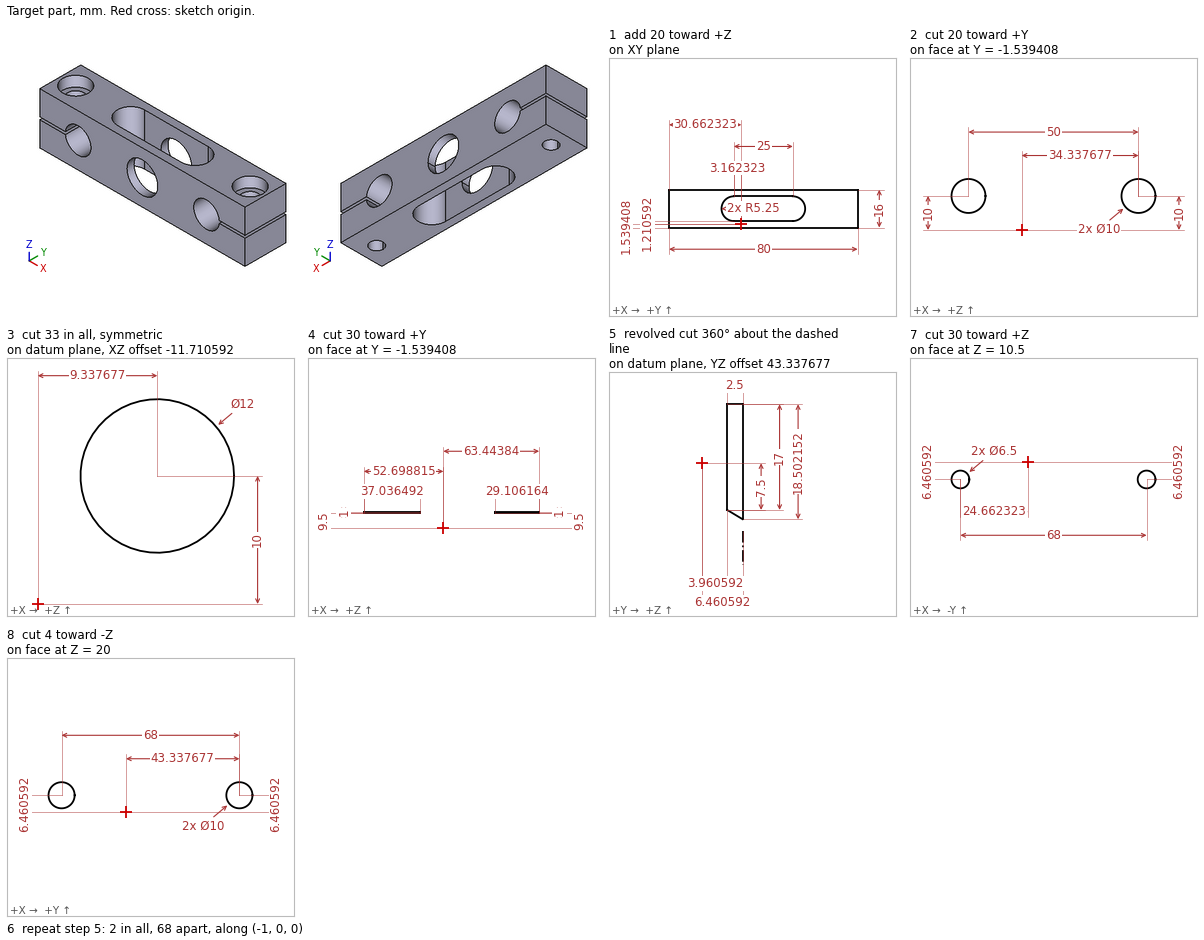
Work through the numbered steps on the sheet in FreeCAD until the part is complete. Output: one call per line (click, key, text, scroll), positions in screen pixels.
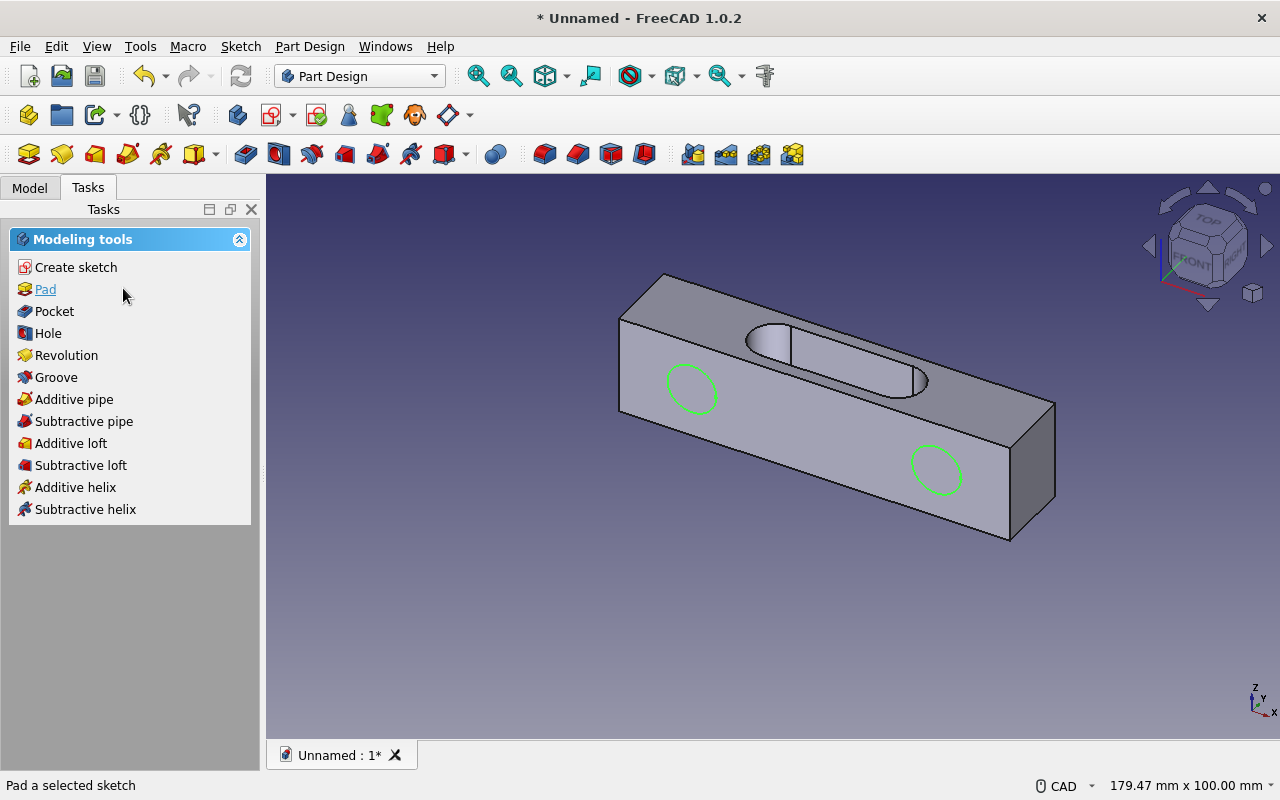
click(246, 154)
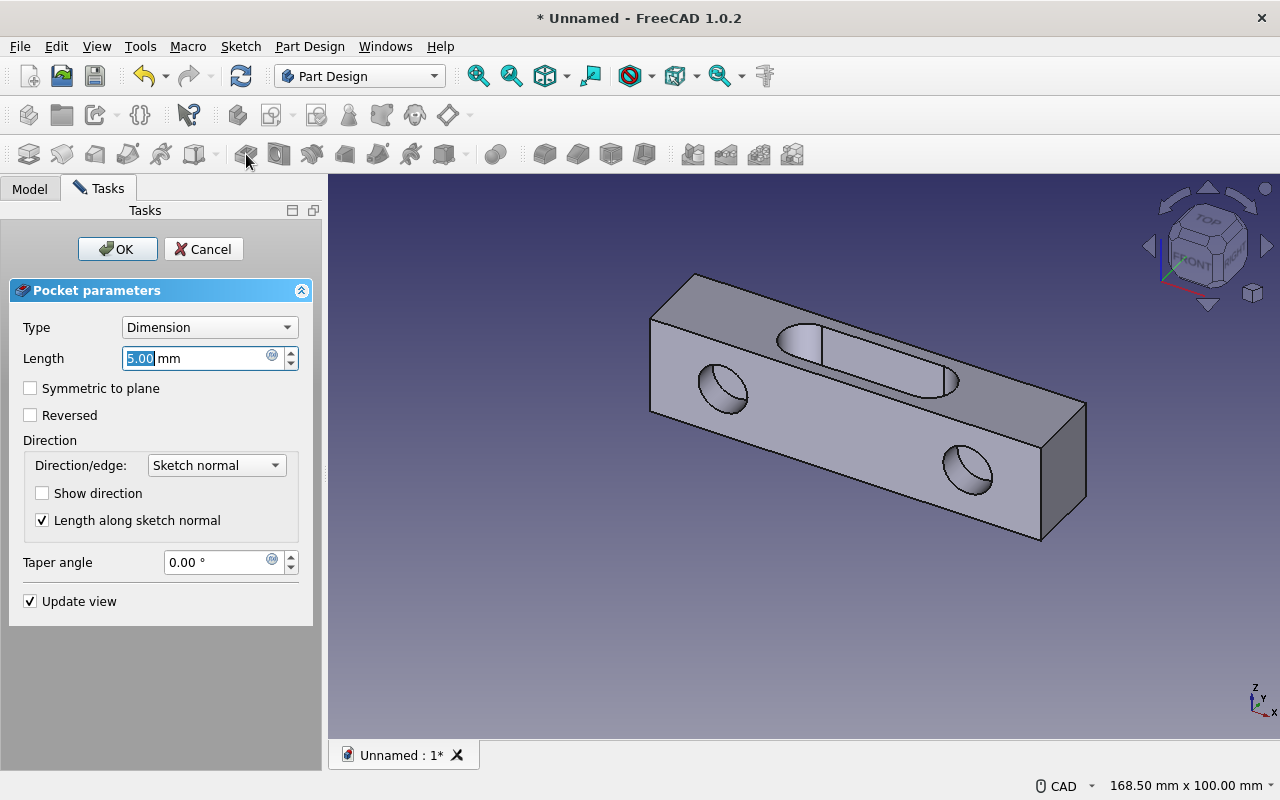
text(20)
key(Tab)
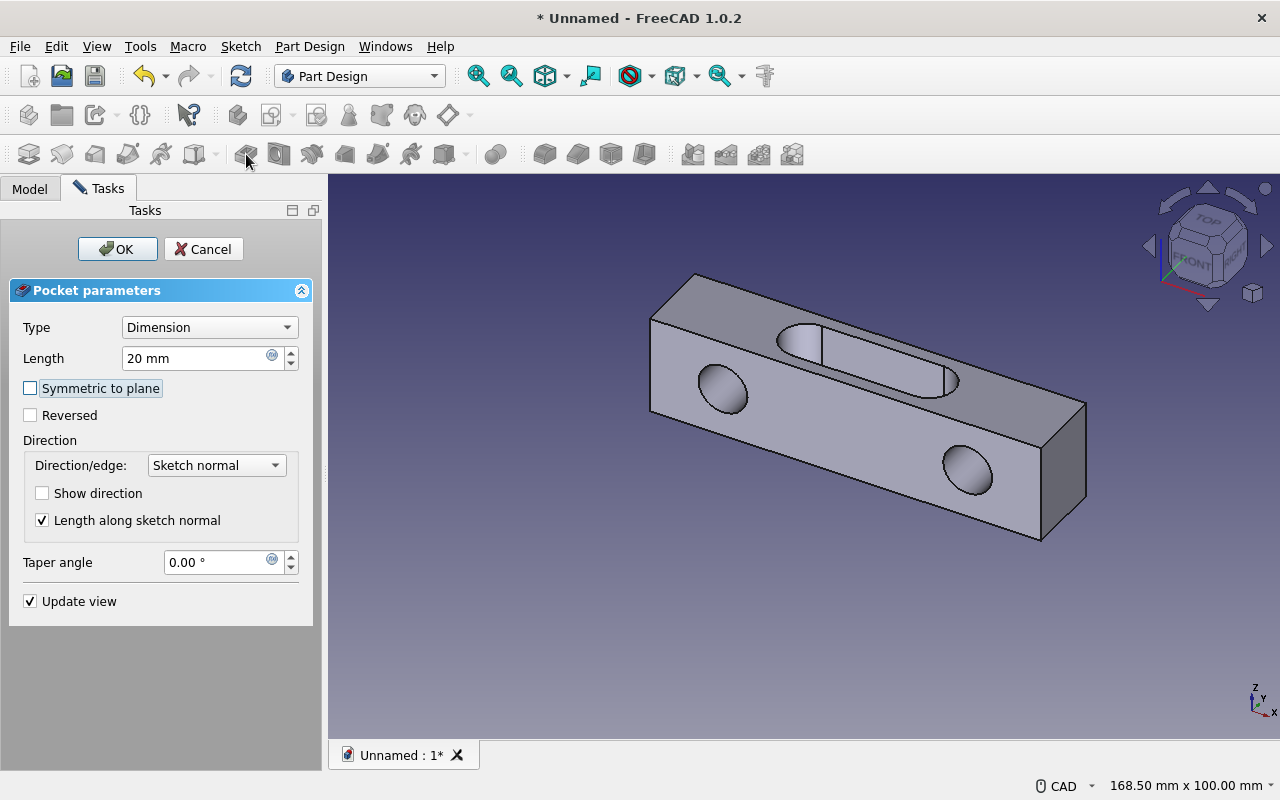
click(118, 249)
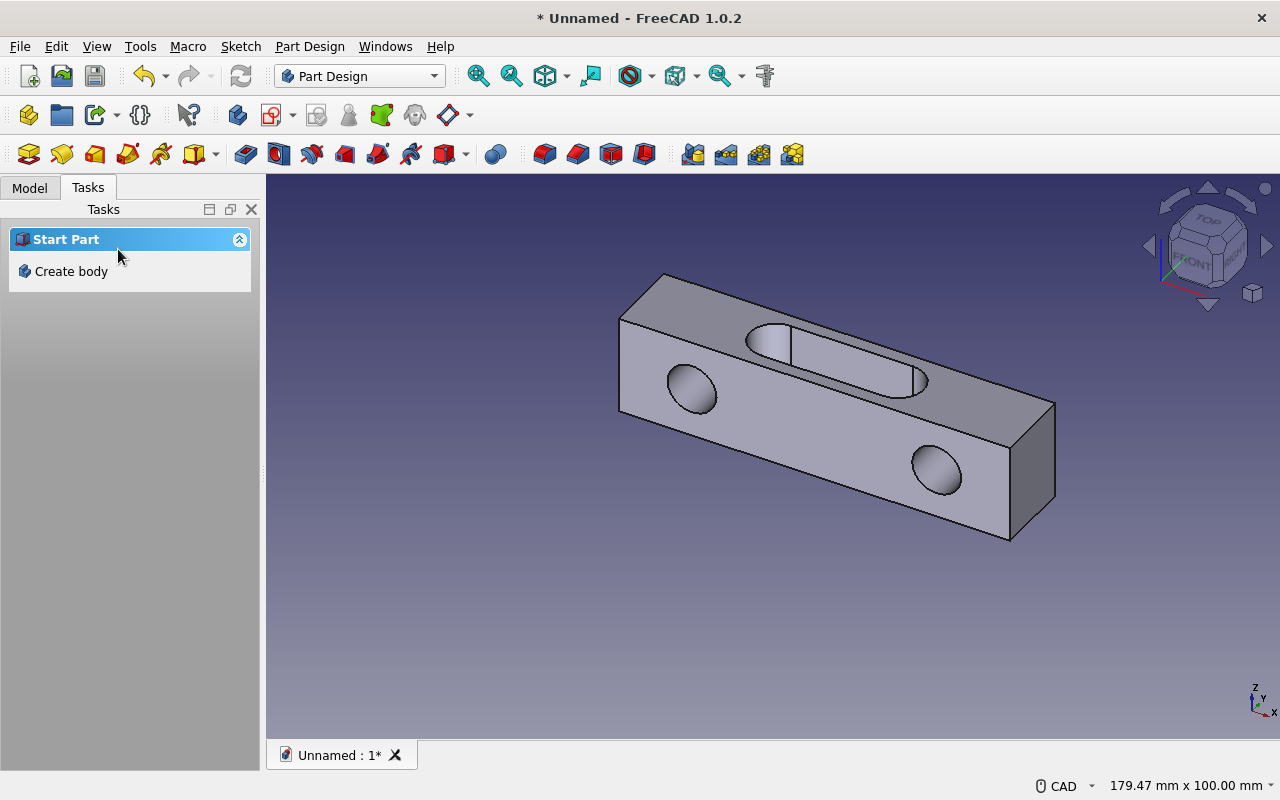
click(30, 188)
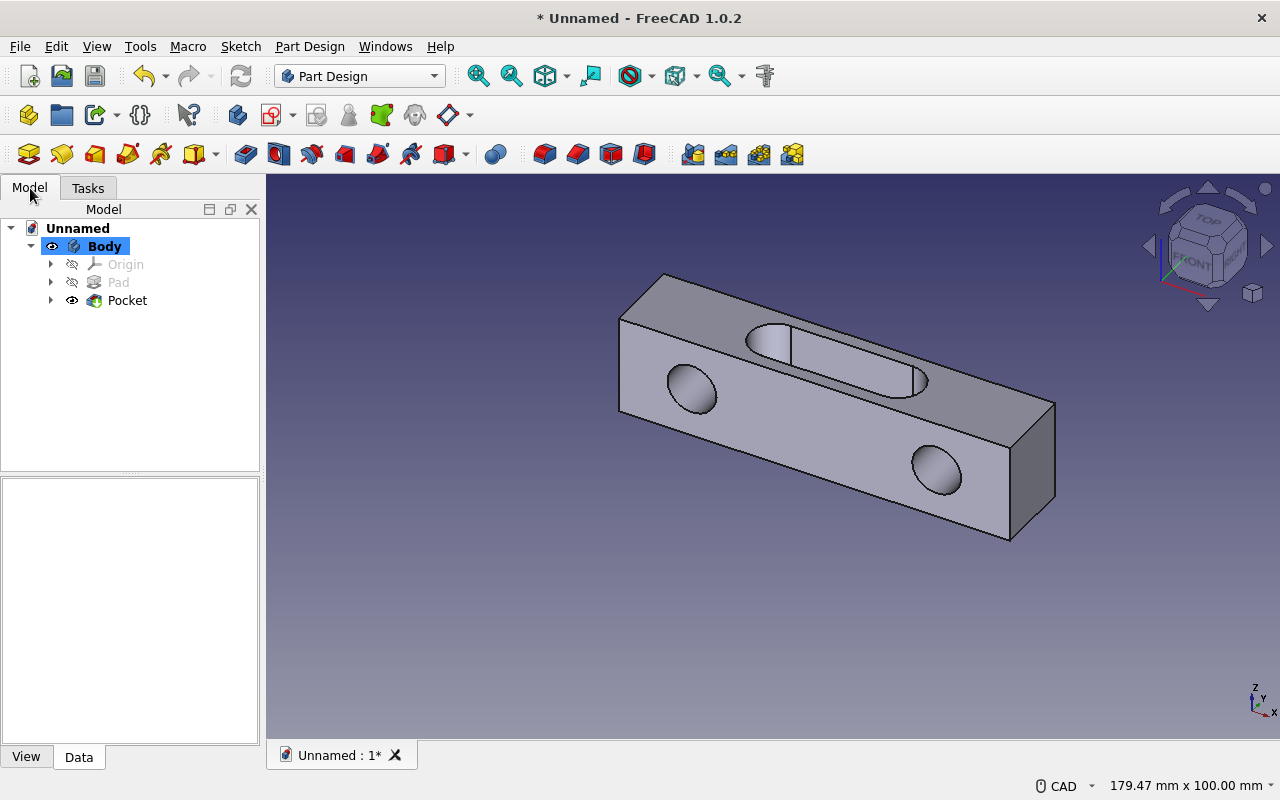
click(51, 264)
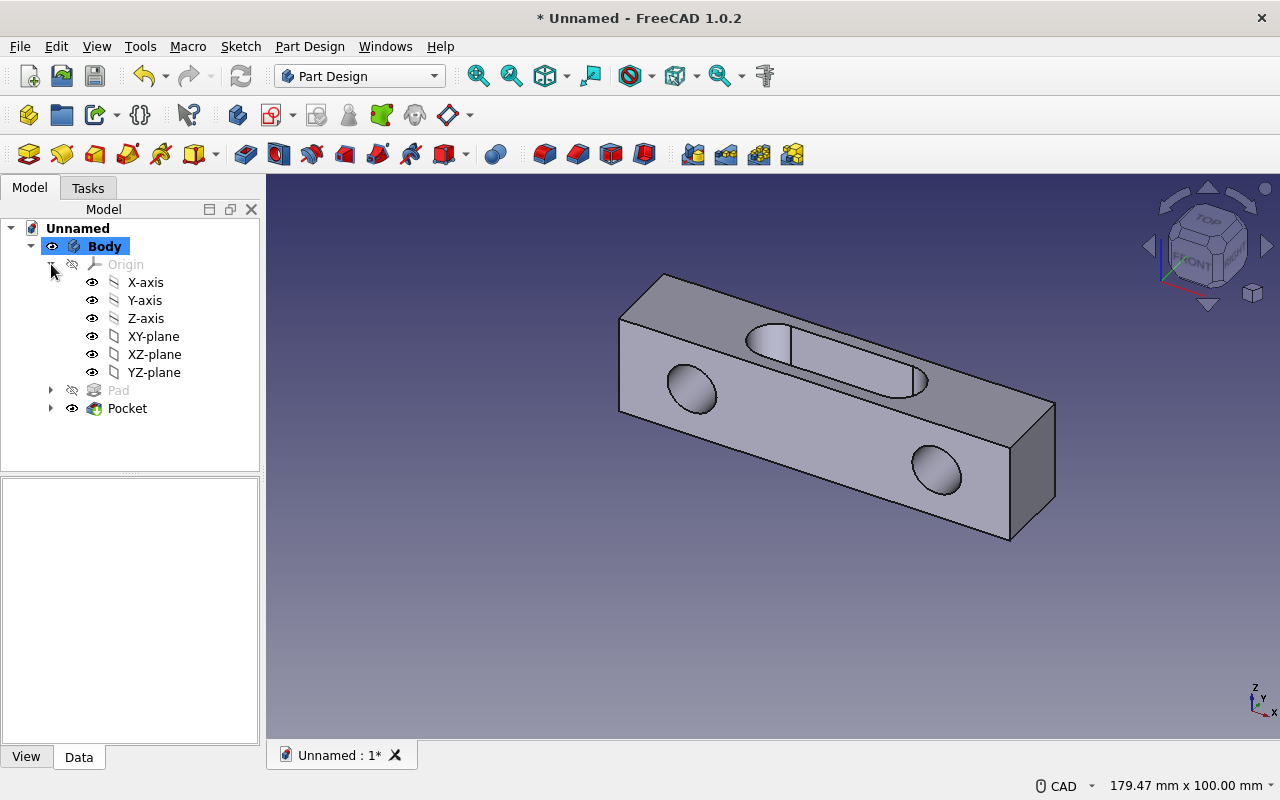
click(137, 354)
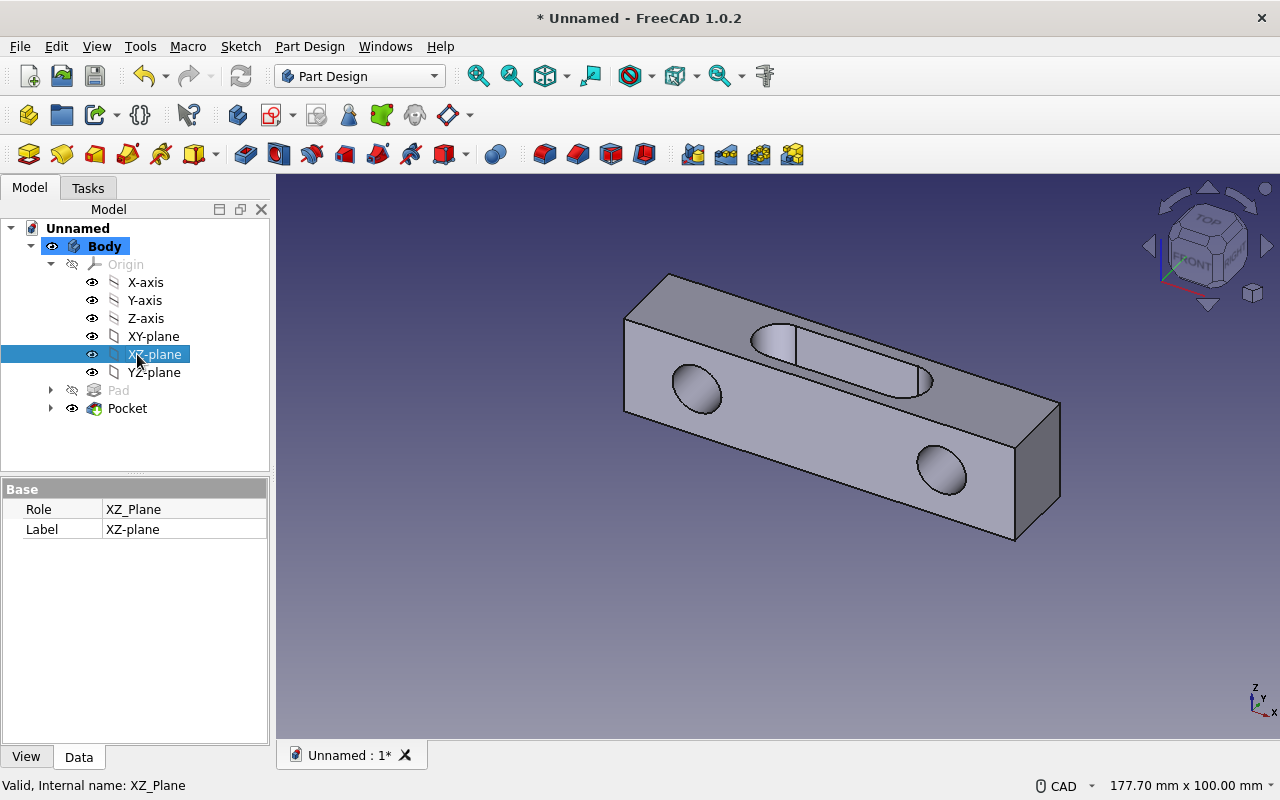
click(448, 116)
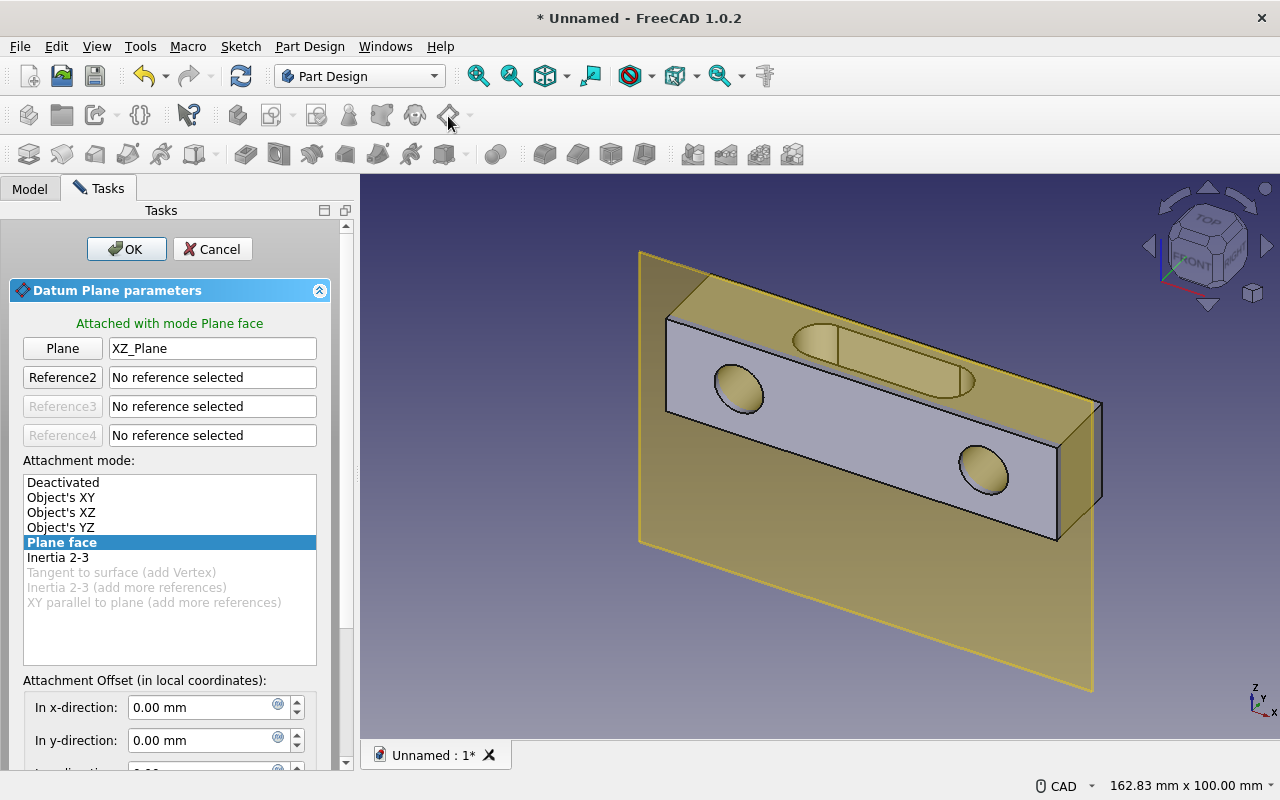
scroll(346, 495, down, 2)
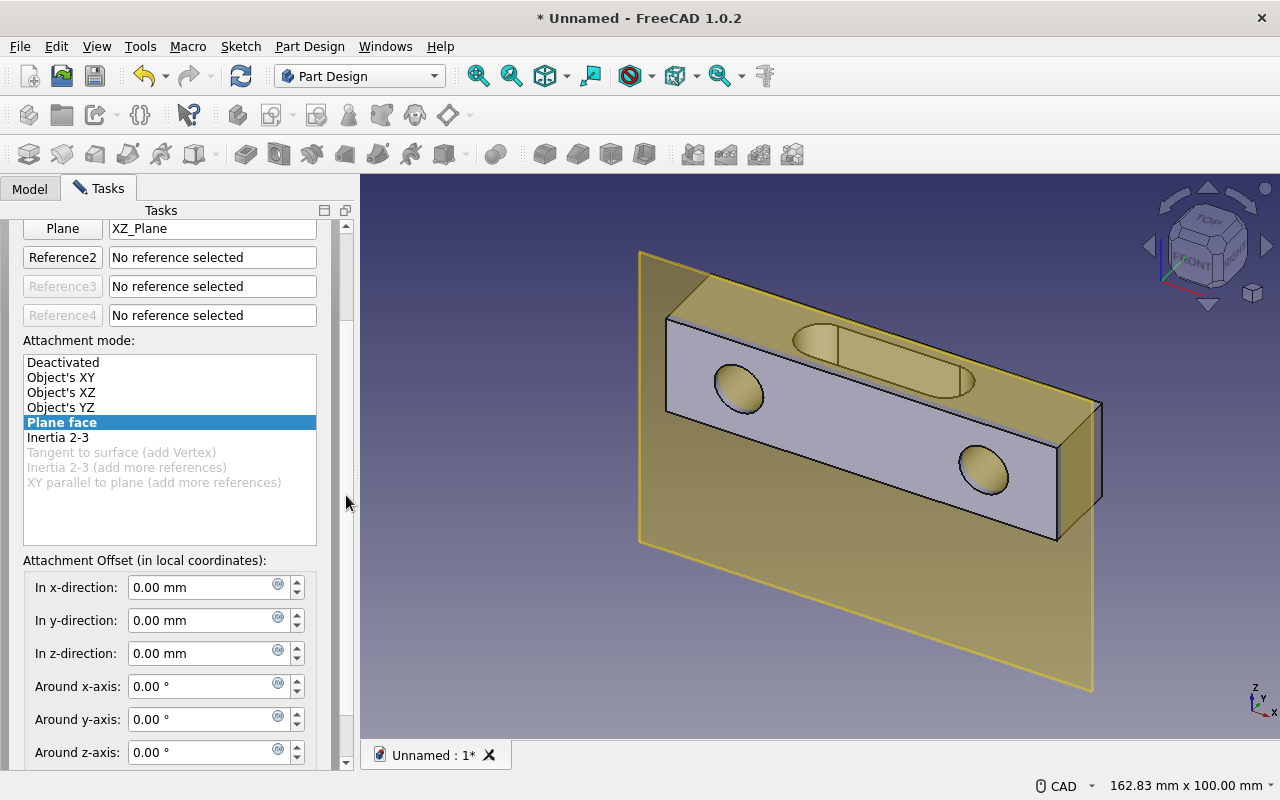
triple_click(210, 654)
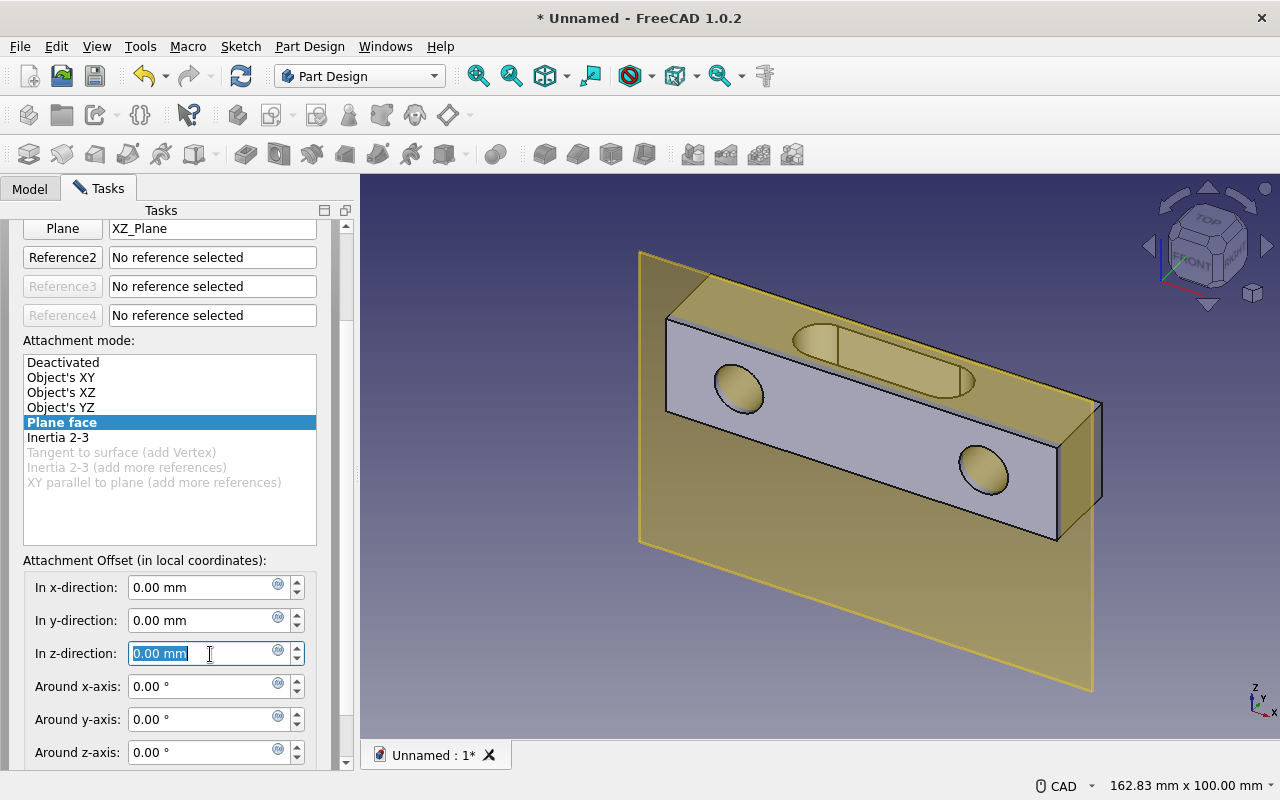
text(-11.710592)
key(Tab)